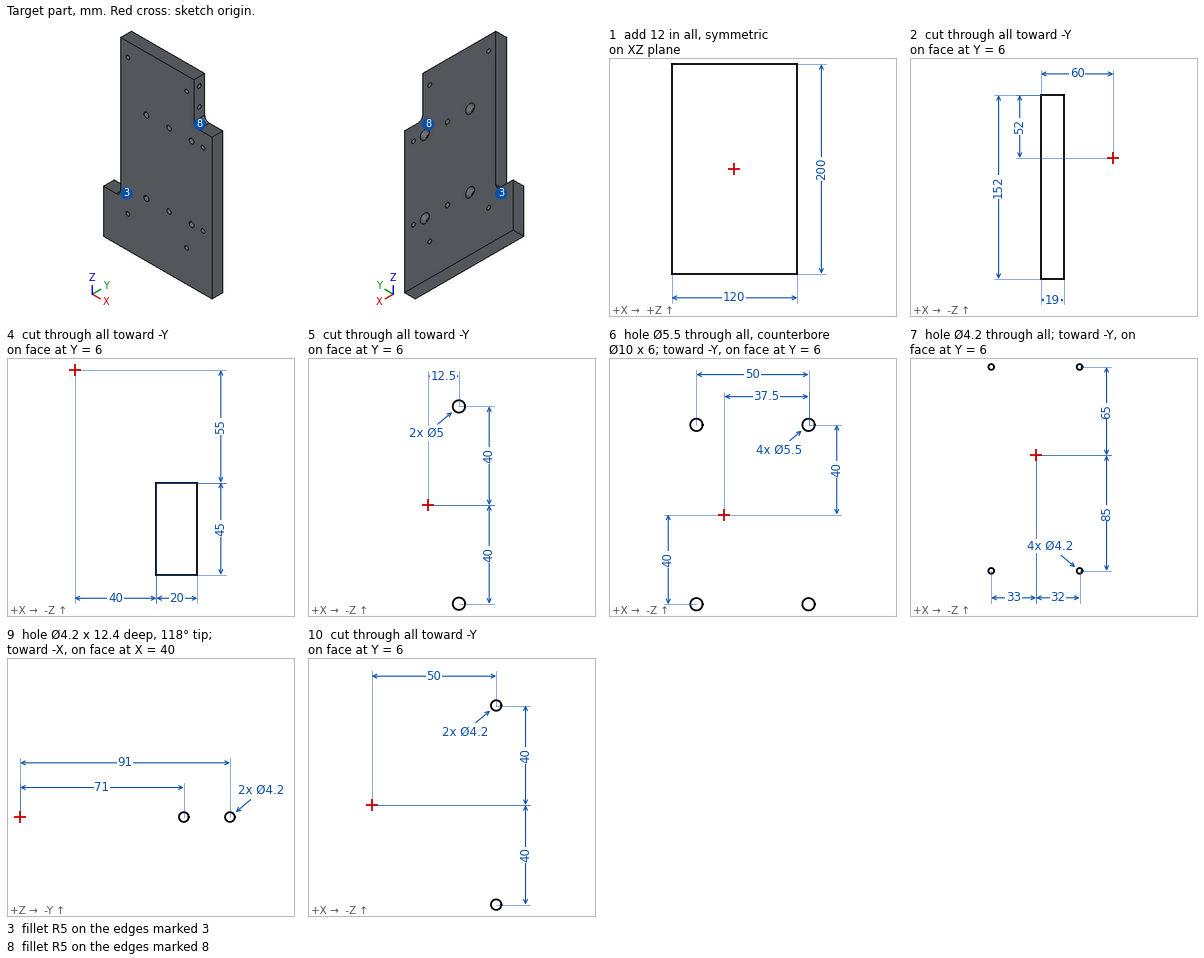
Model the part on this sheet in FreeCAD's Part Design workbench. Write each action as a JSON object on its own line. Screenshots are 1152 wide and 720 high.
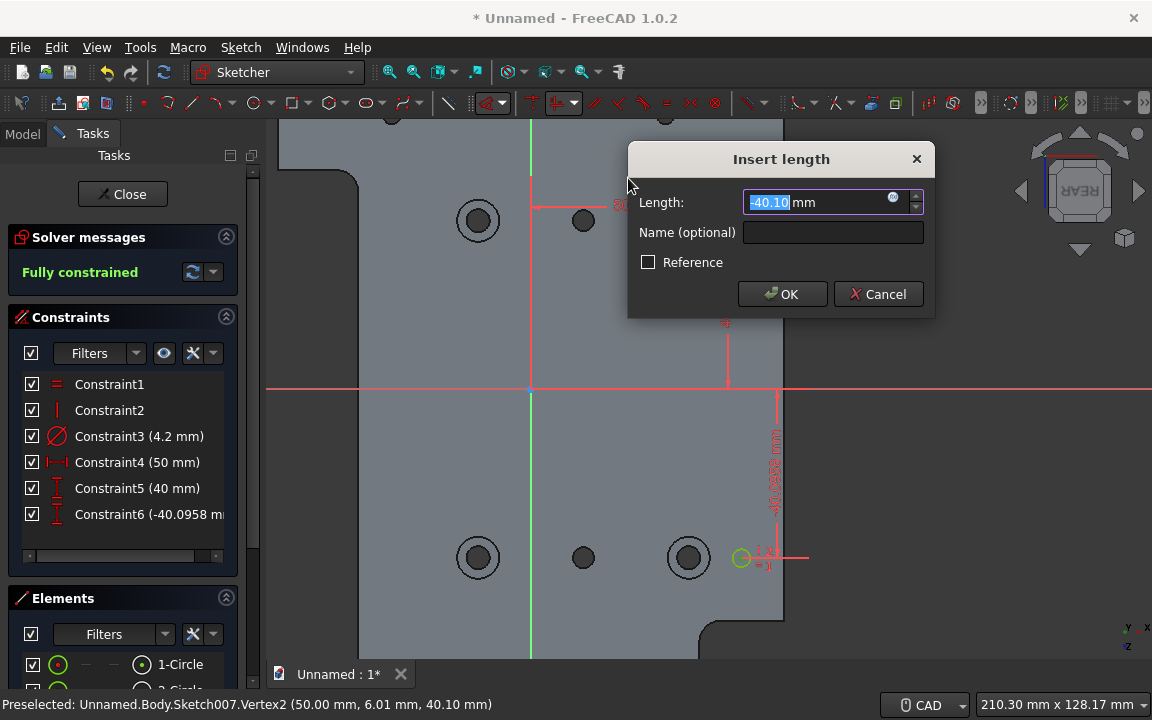
{"action": "type", "text": "-40"}
{"action": "key", "text": "Return"}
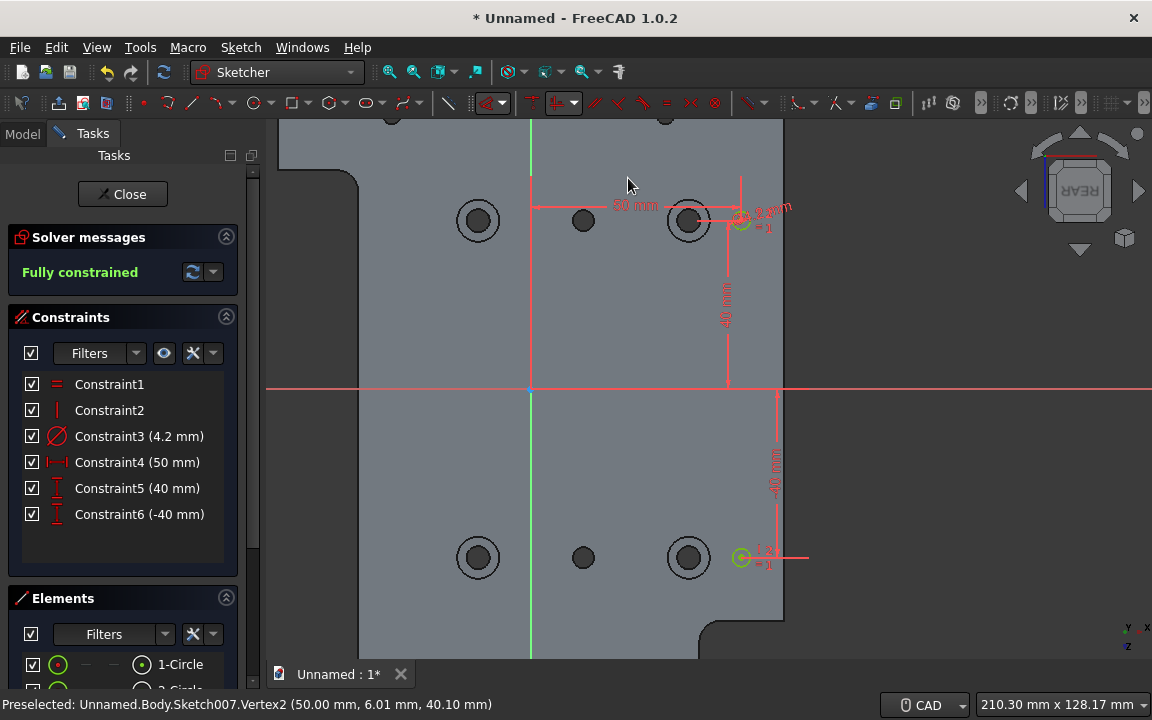
{"action": "left_click", "coordinate": [123, 194]}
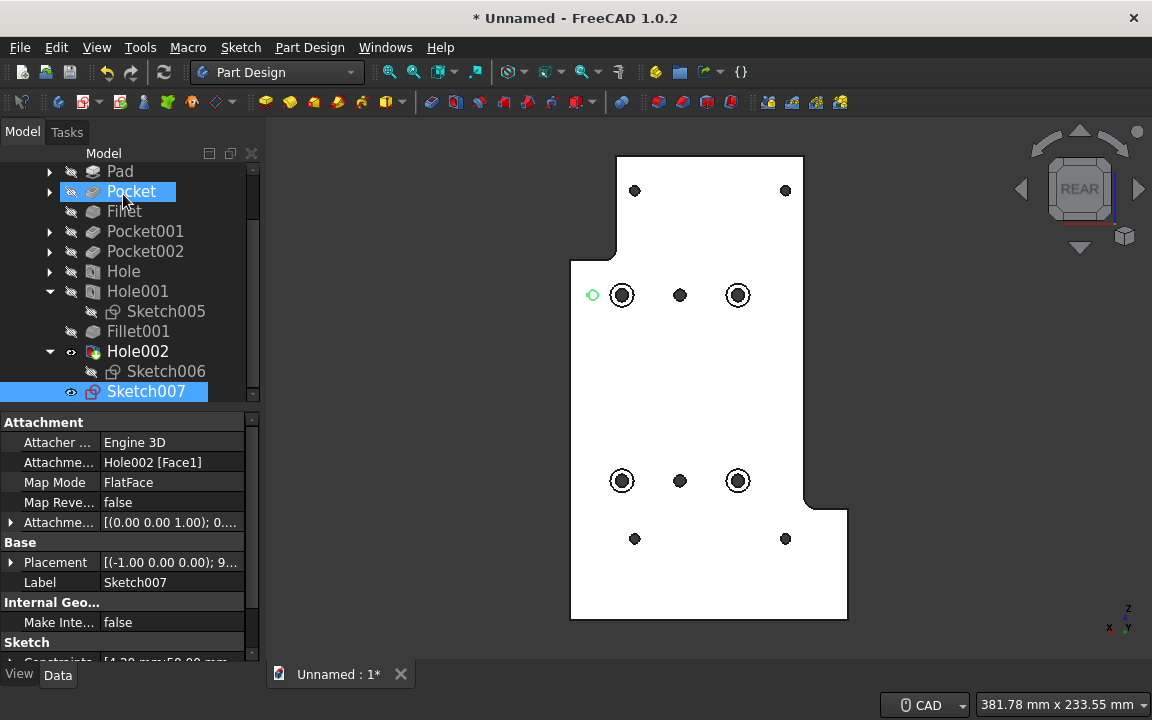
{"action": "left_click", "coordinate": [432, 102]}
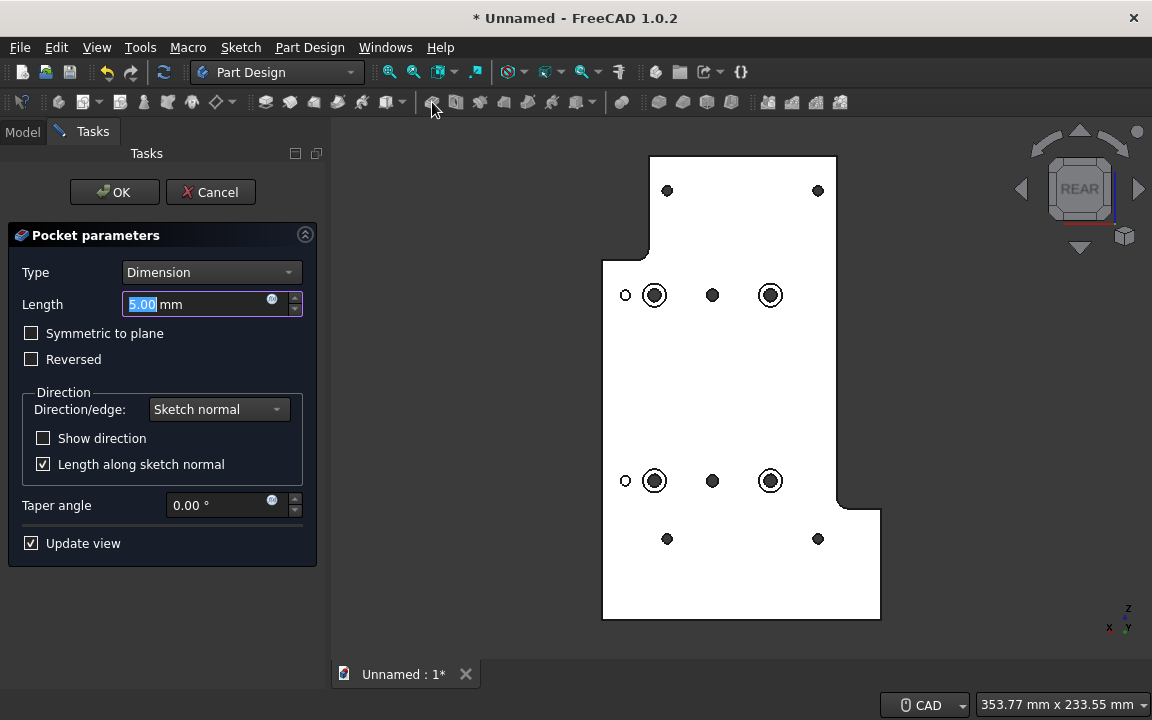
{"action": "left_click", "coordinate": [212, 272]}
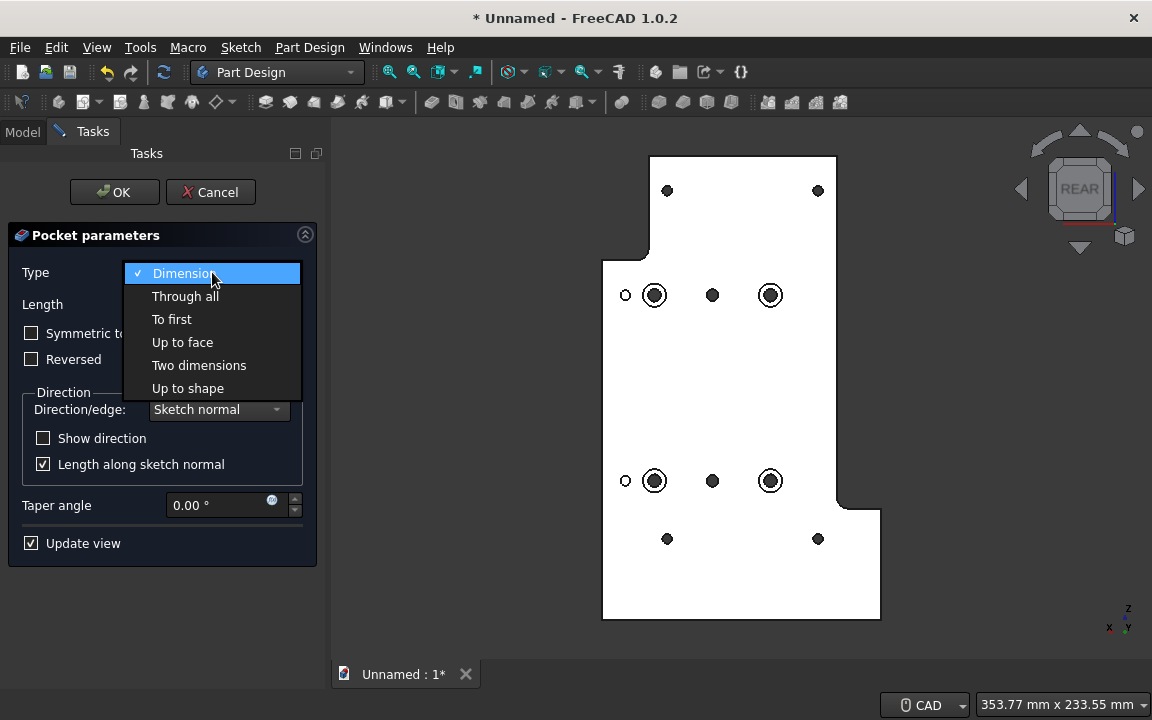
{"action": "left_click", "coordinate": [212, 296]}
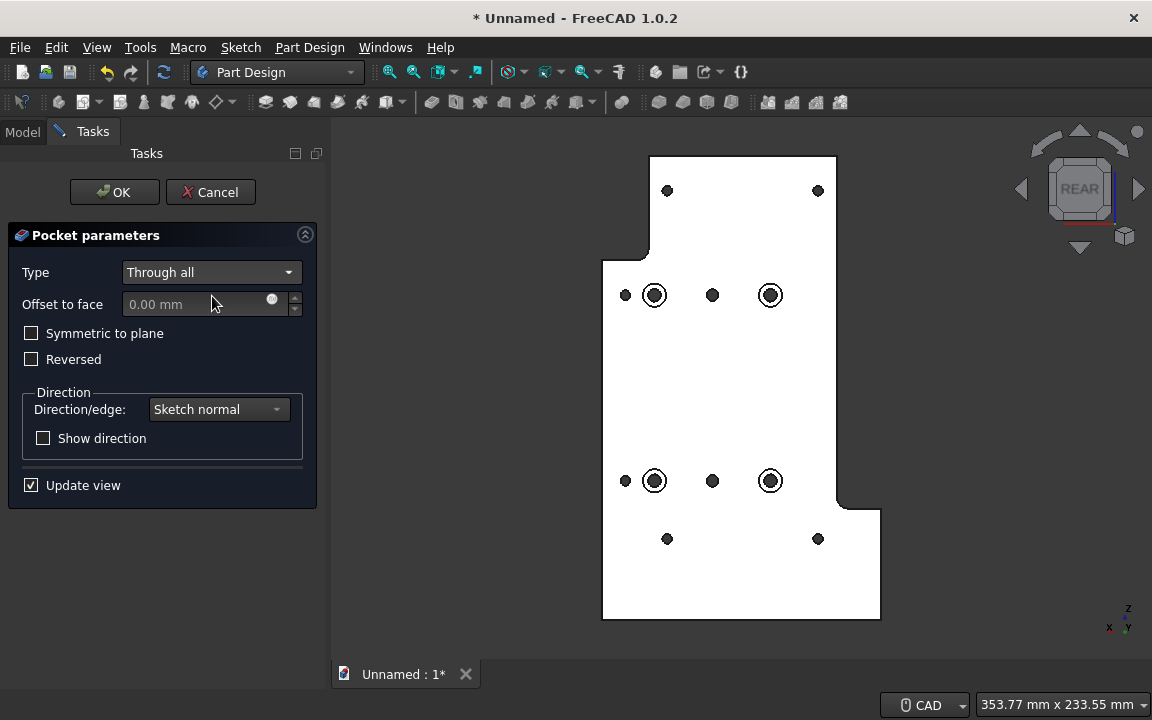
{"action": "left_click", "coordinate": [115, 192]}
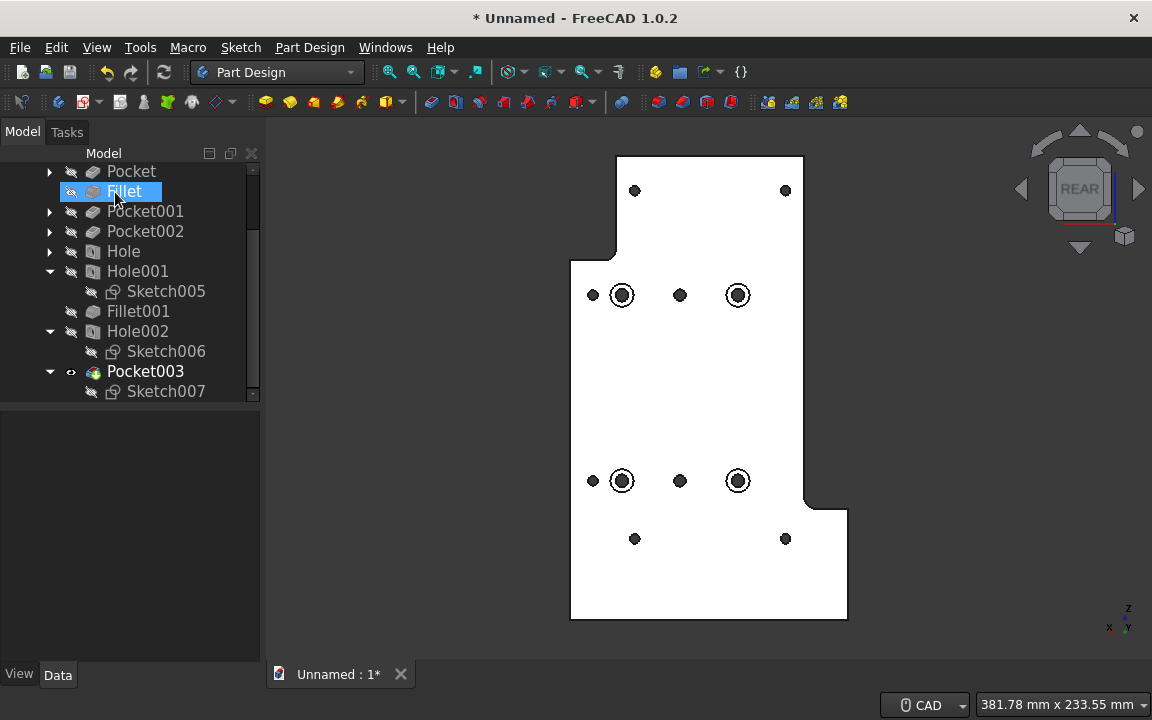
{"action": "key", "text": "0"}